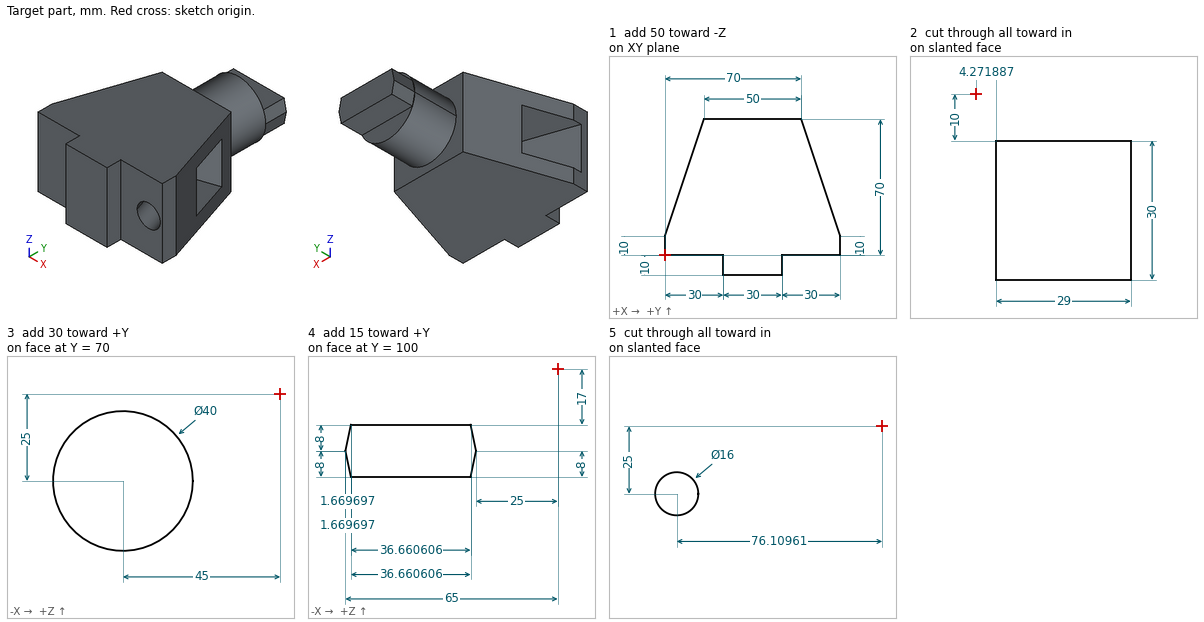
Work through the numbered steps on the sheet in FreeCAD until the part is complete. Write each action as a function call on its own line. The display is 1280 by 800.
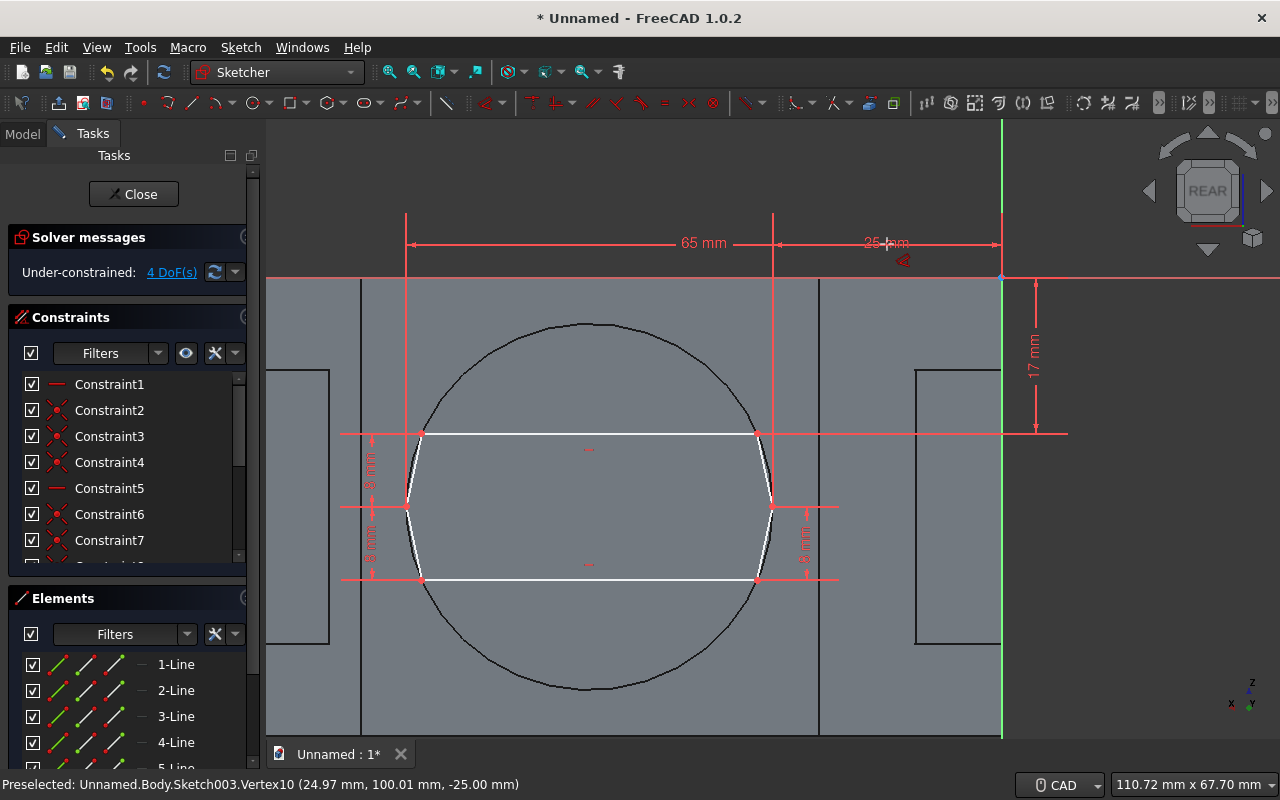
click(657, 434)
click(590, 468)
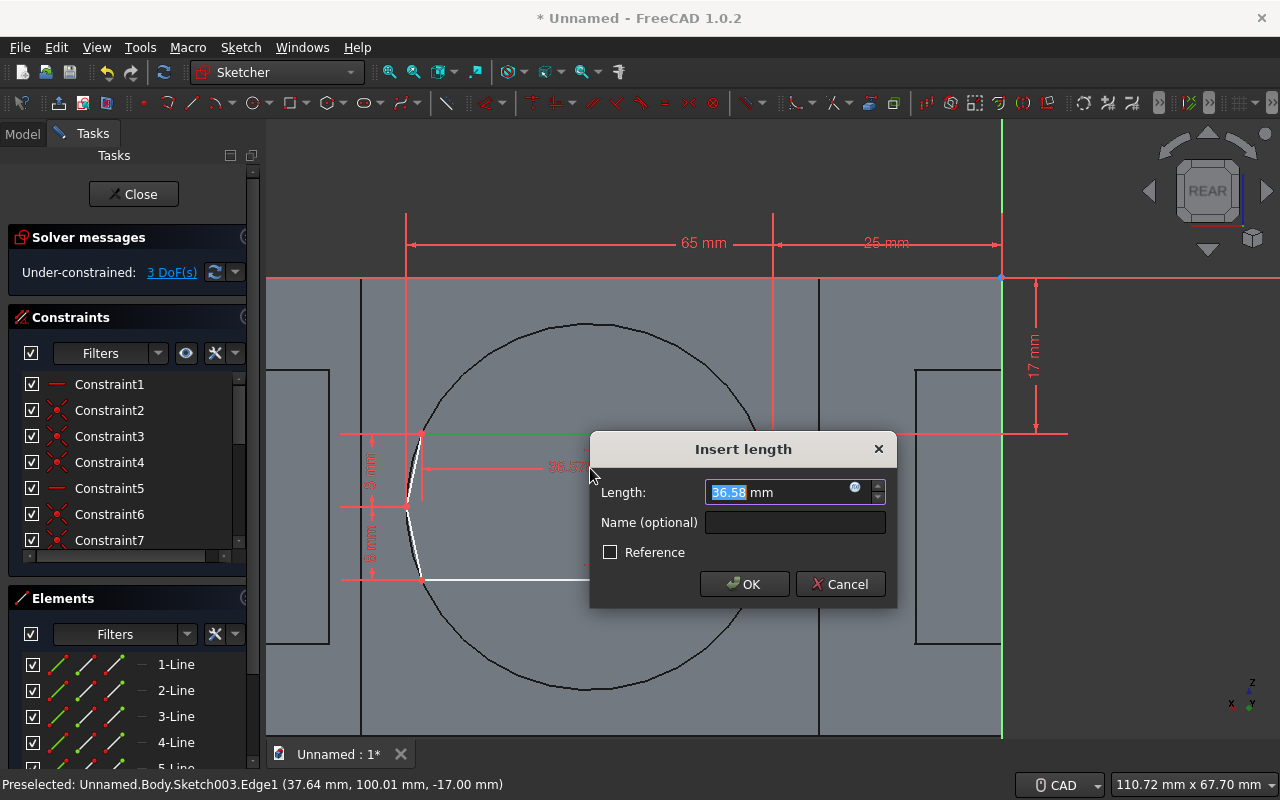
text(36.660606)
key(Return)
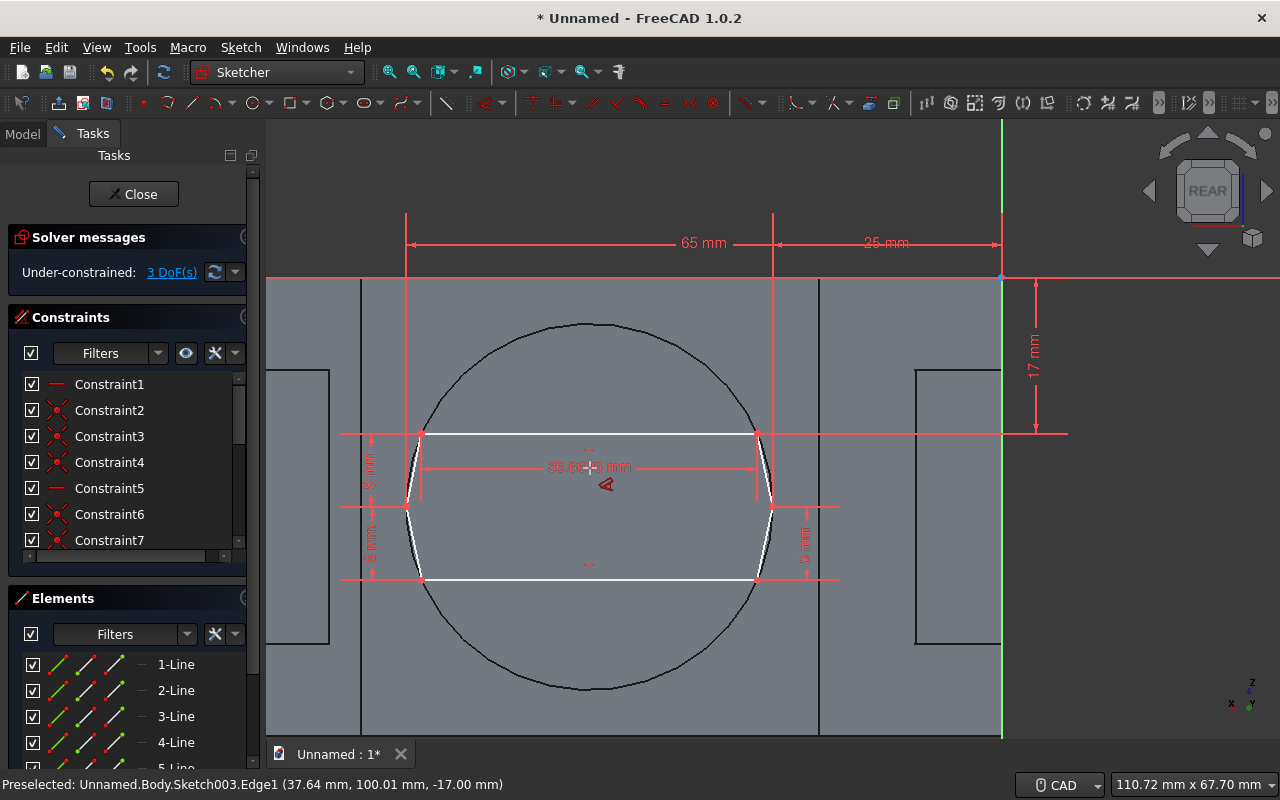
click(523, 580)
click(590, 614)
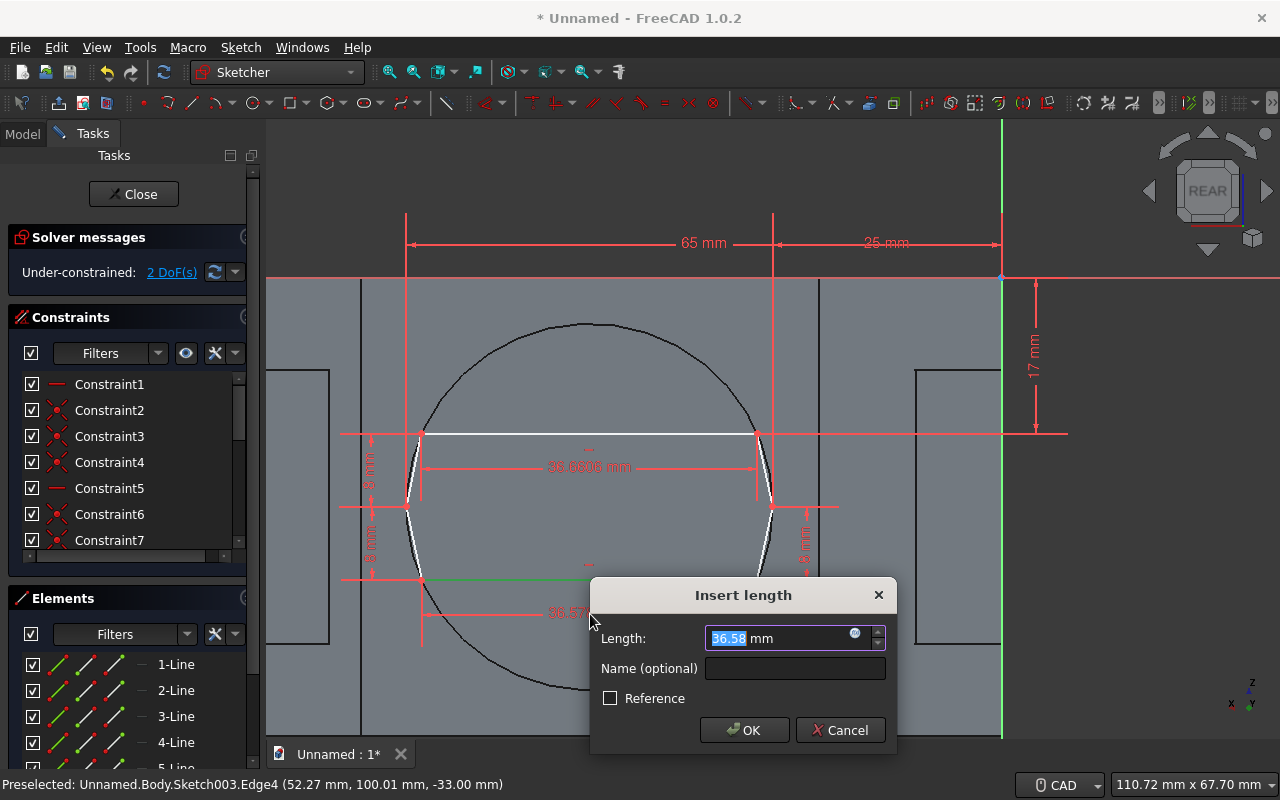
text(36.660606)
key(Return)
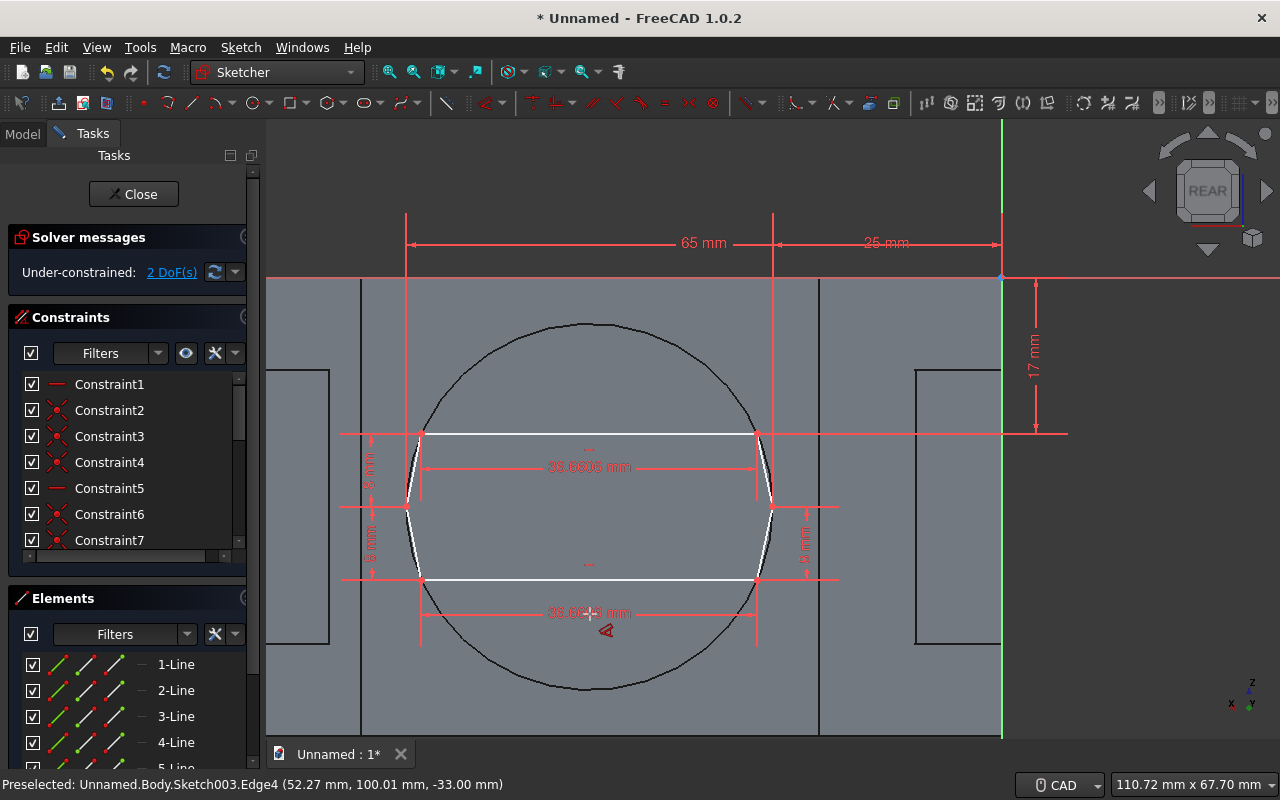
scroll(417, 456, up, 5)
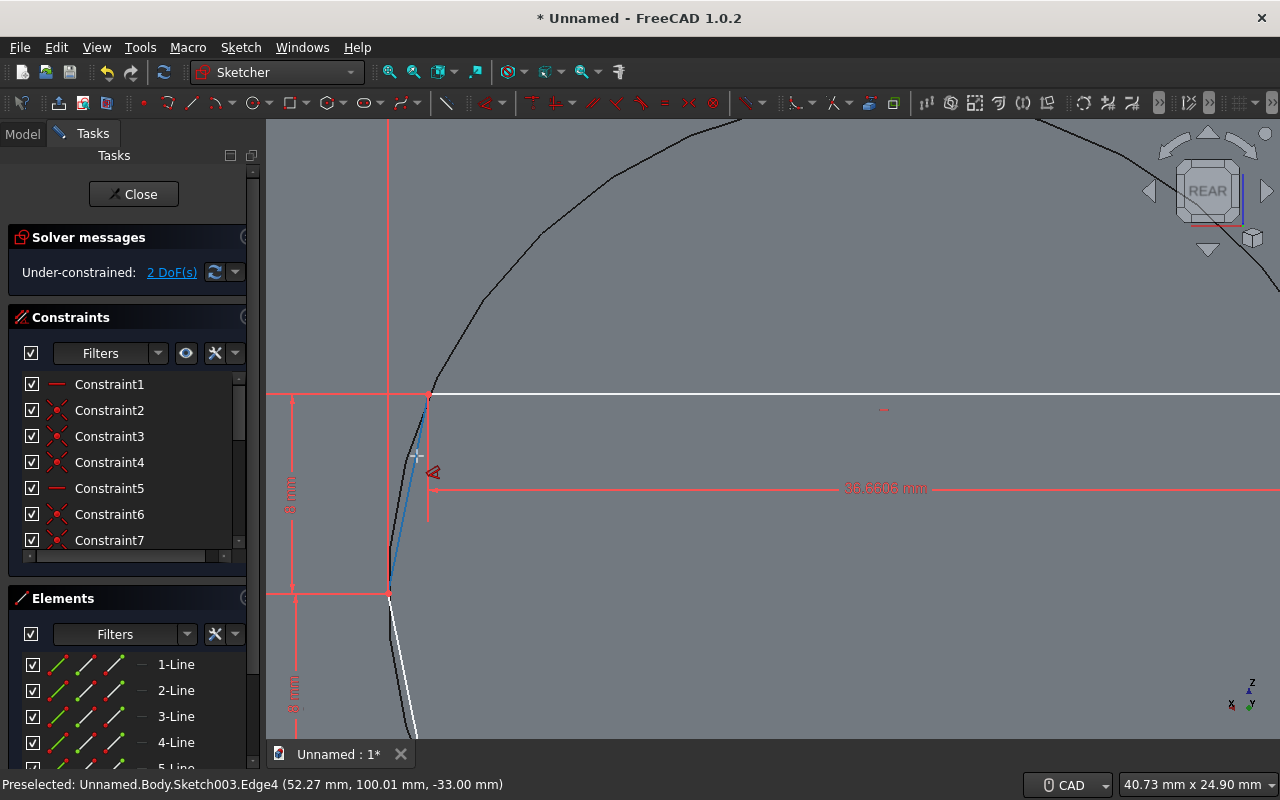
click(416, 454)
click(417, 628)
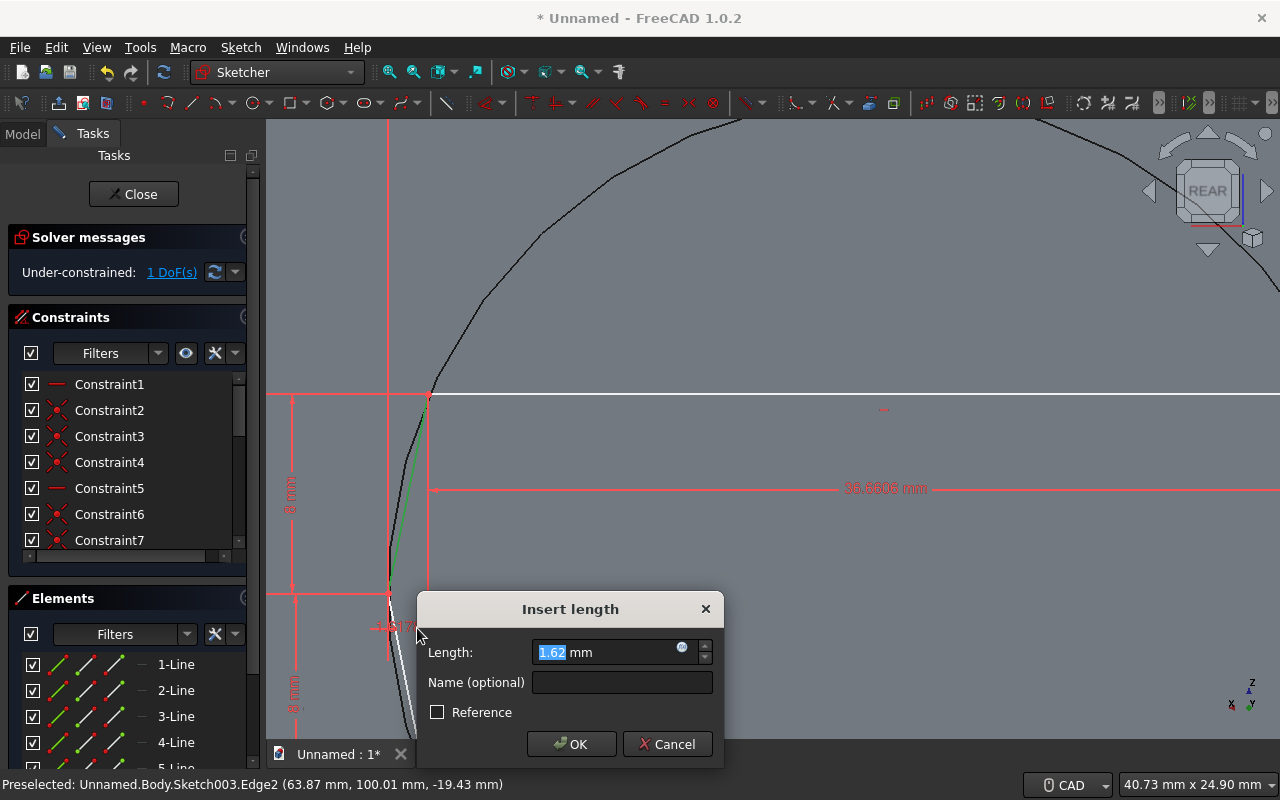
text(1.669697)
key(Return)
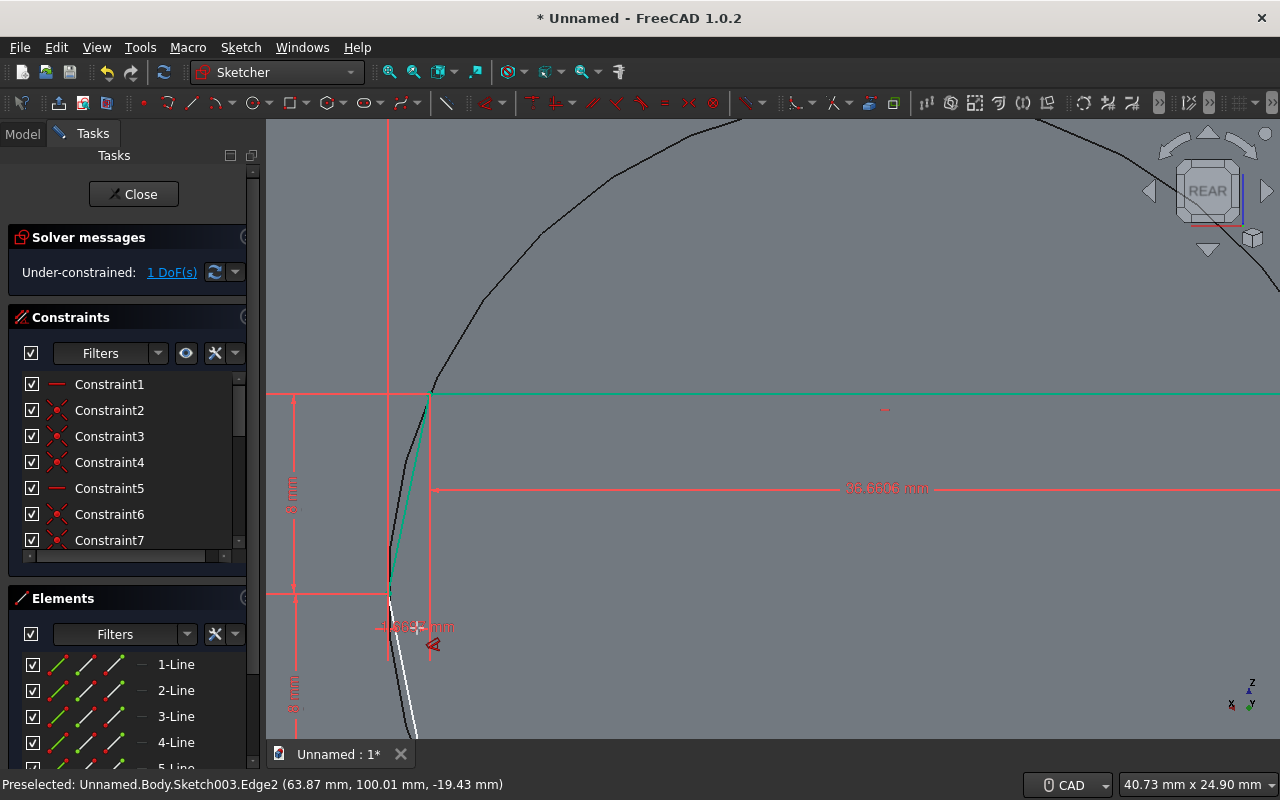
click(400, 653)
click(417, 560)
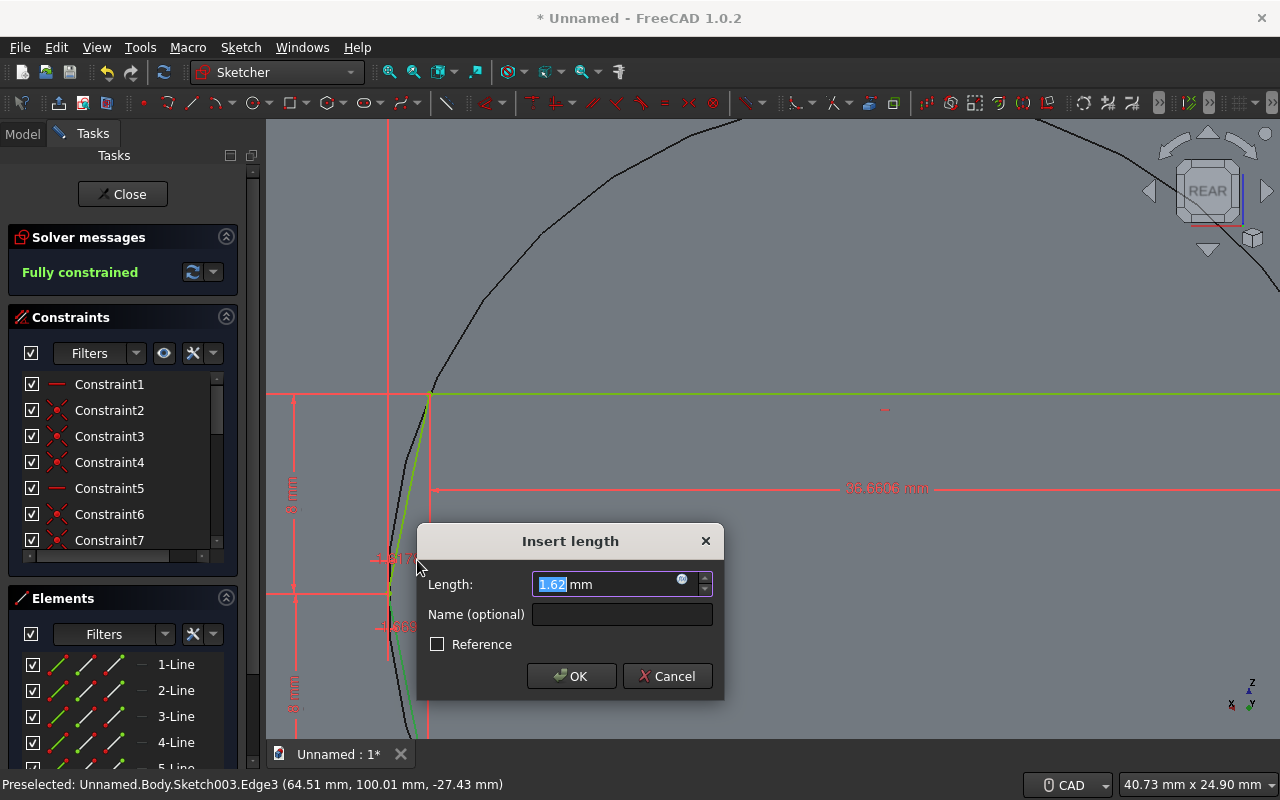
text(1.669697)
key(Return)
key(Escape)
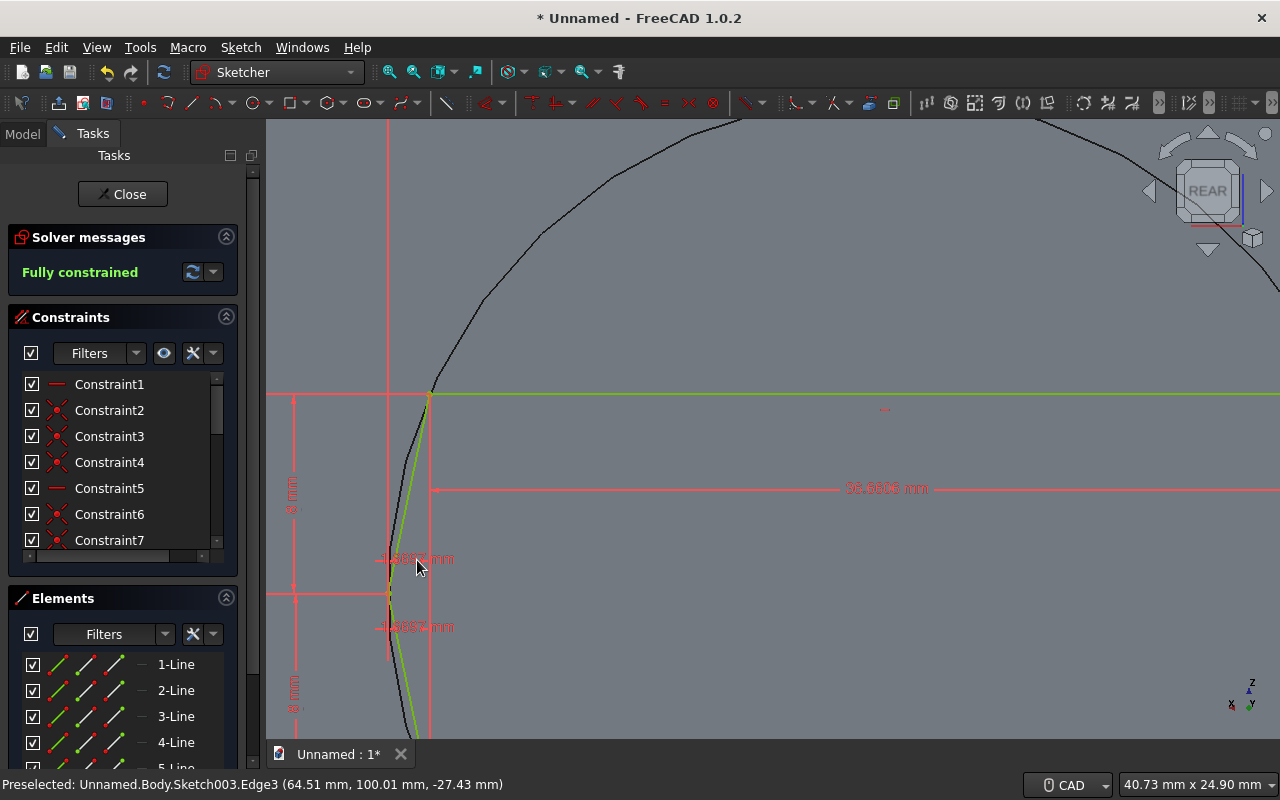
click(123, 194)